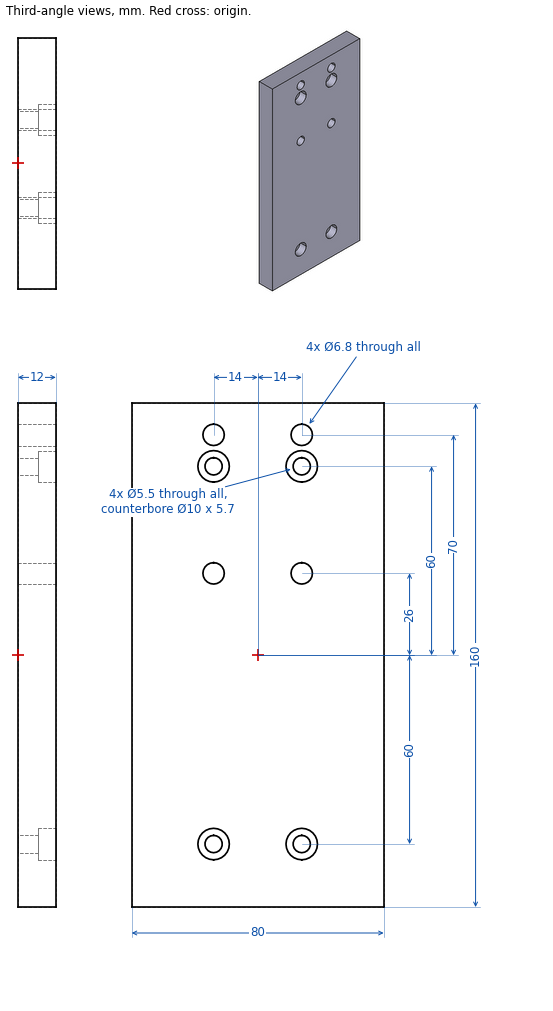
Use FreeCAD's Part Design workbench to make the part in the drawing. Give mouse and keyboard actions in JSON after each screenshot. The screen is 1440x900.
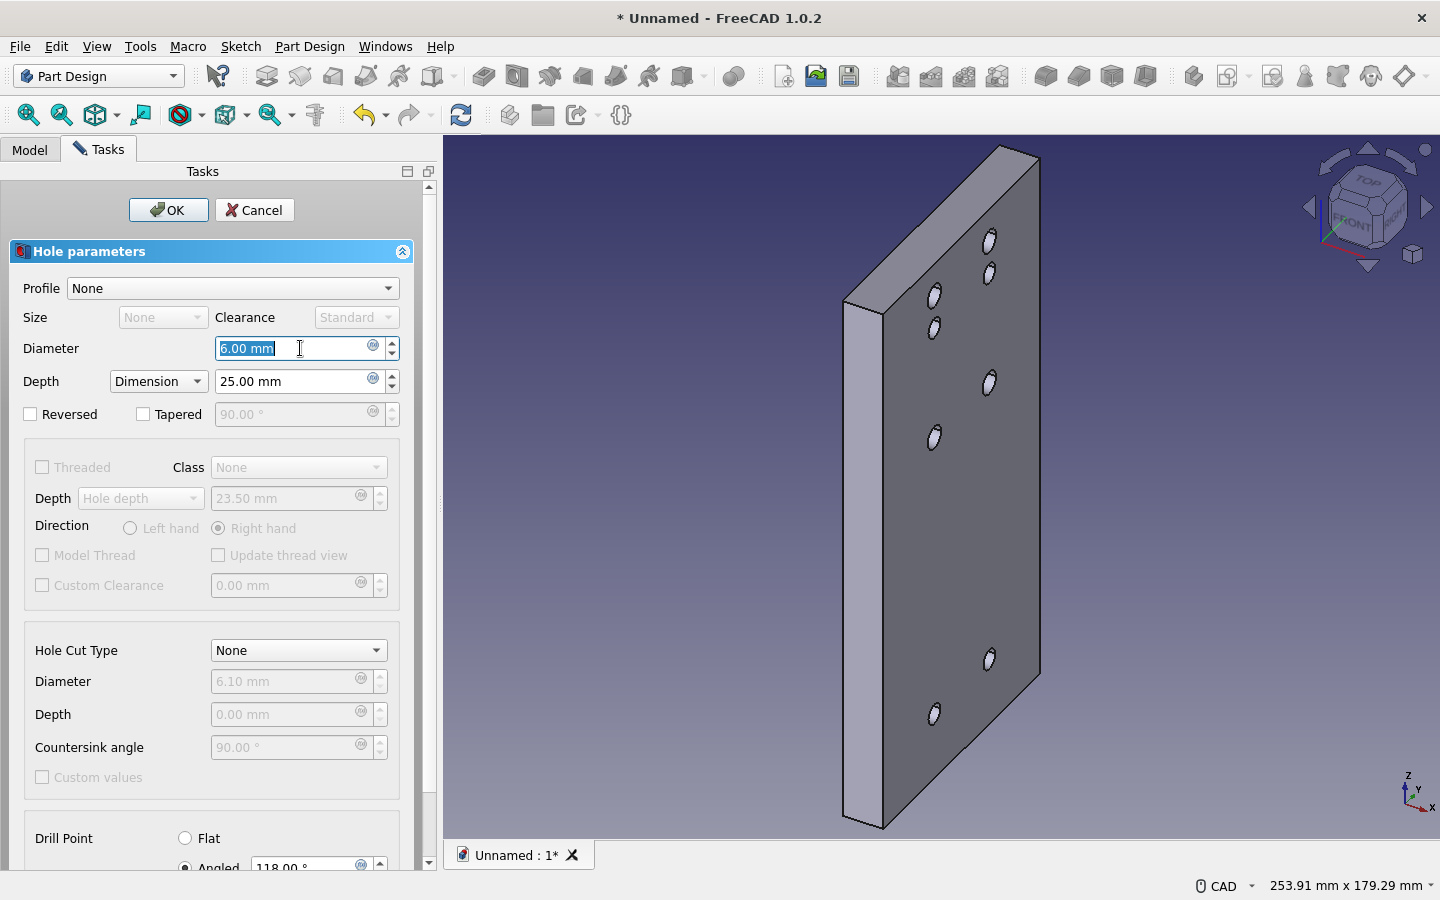
{"action": "type", "text": "5.5"}
{"action": "key", "text": "Tab"}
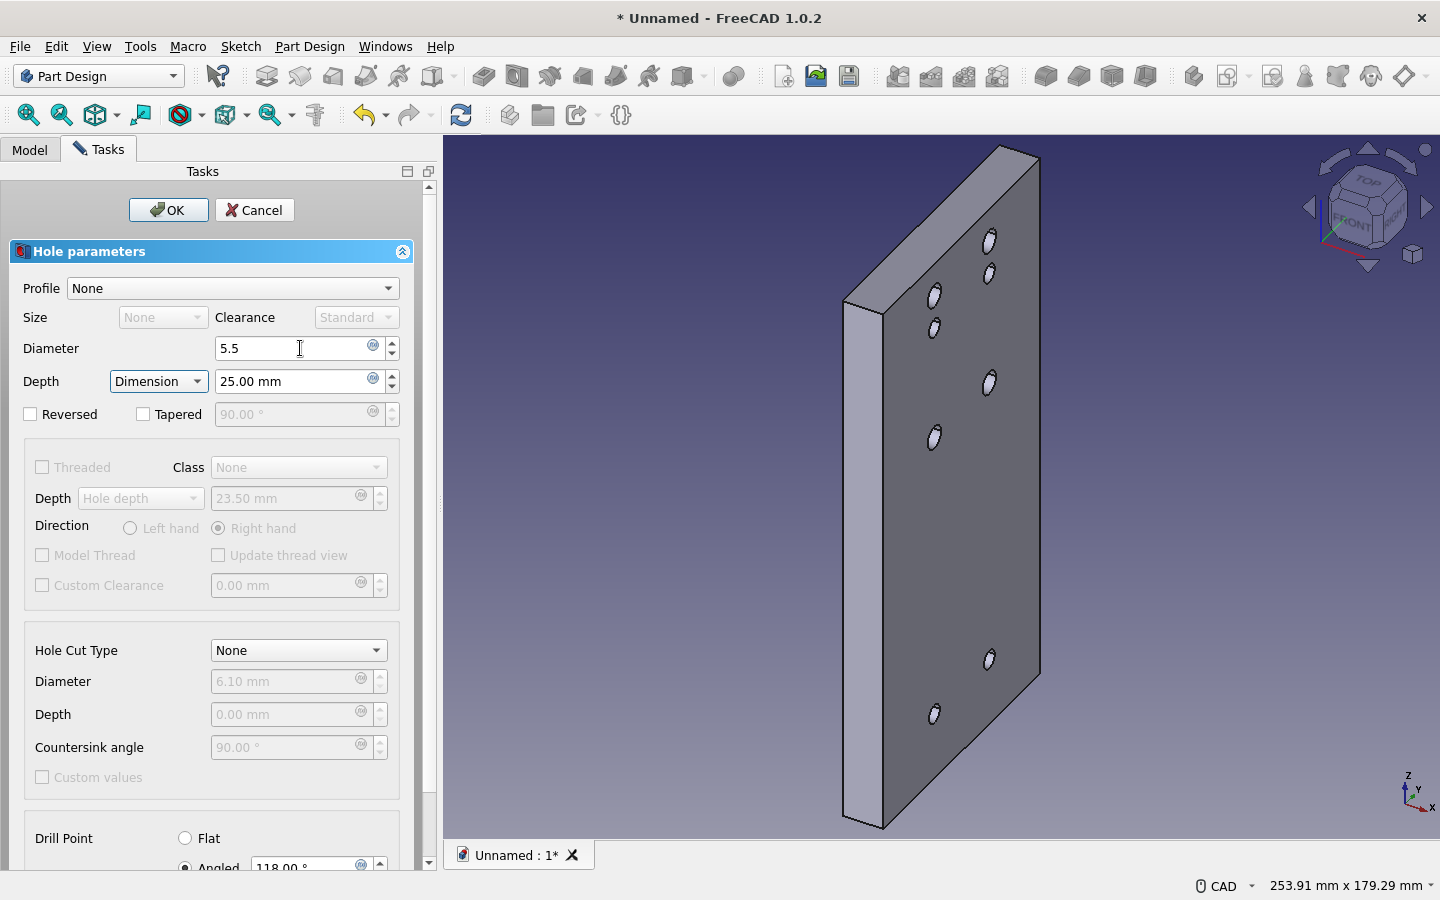
{"action": "left_click", "coordinate": [160, 382]}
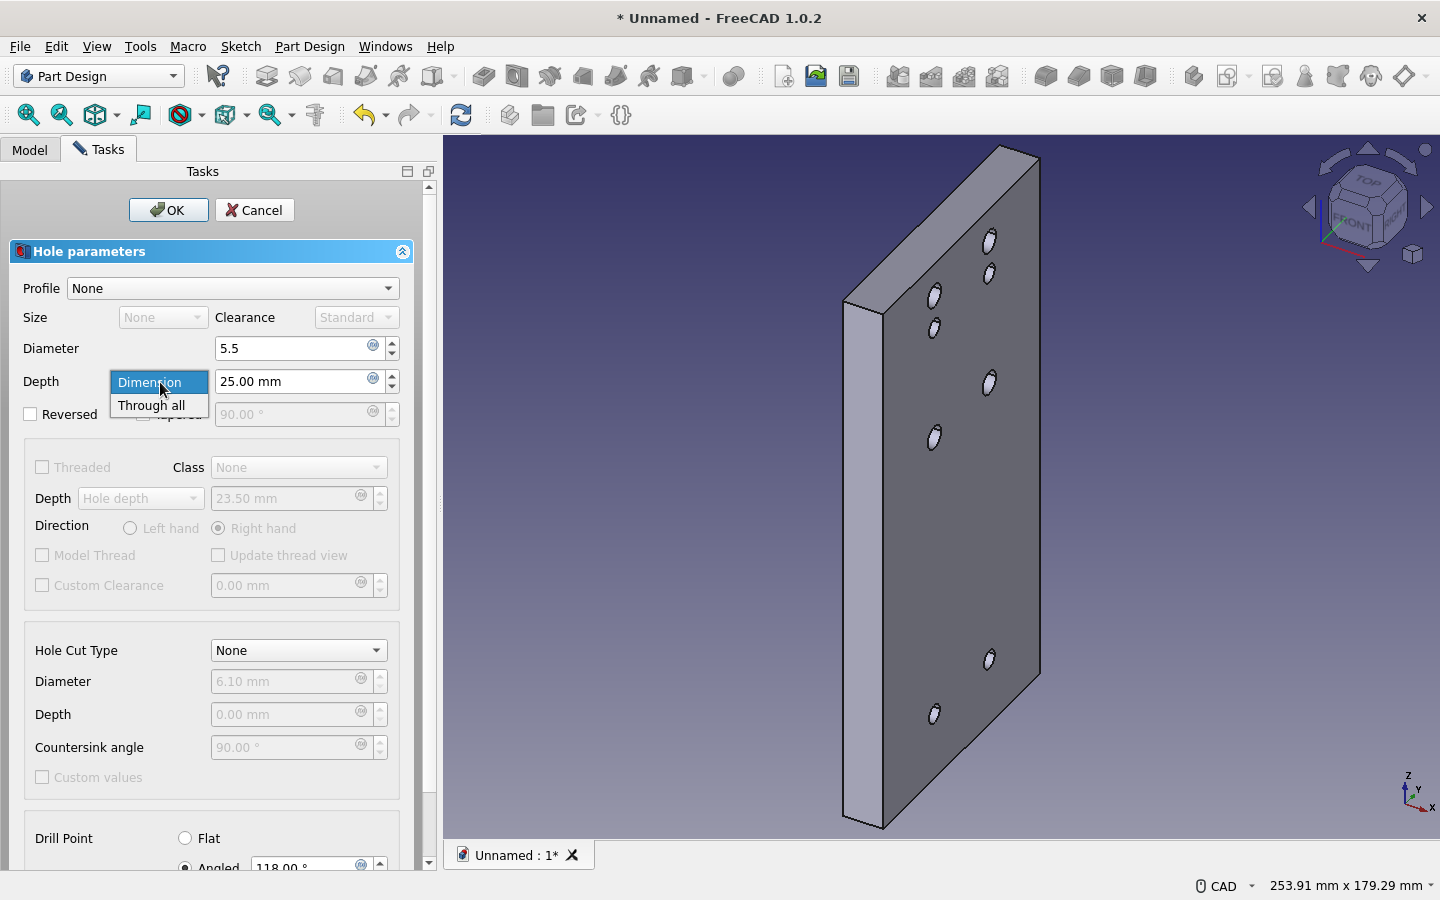
{"action": "left_click", "coordinate": [158, 406]}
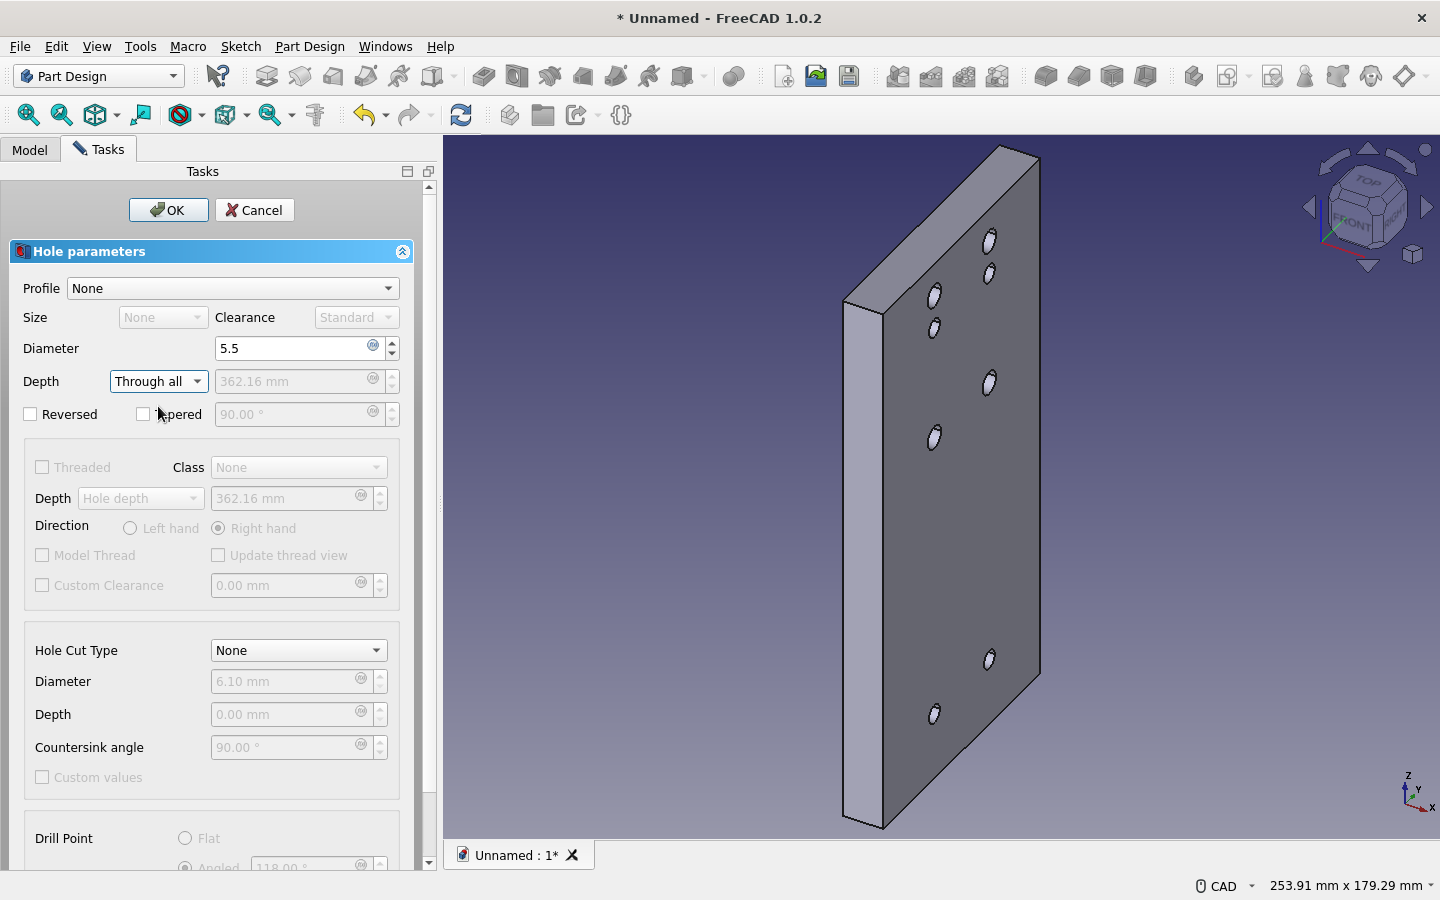
{"action": "left_click", "coordinate": [300, 650]}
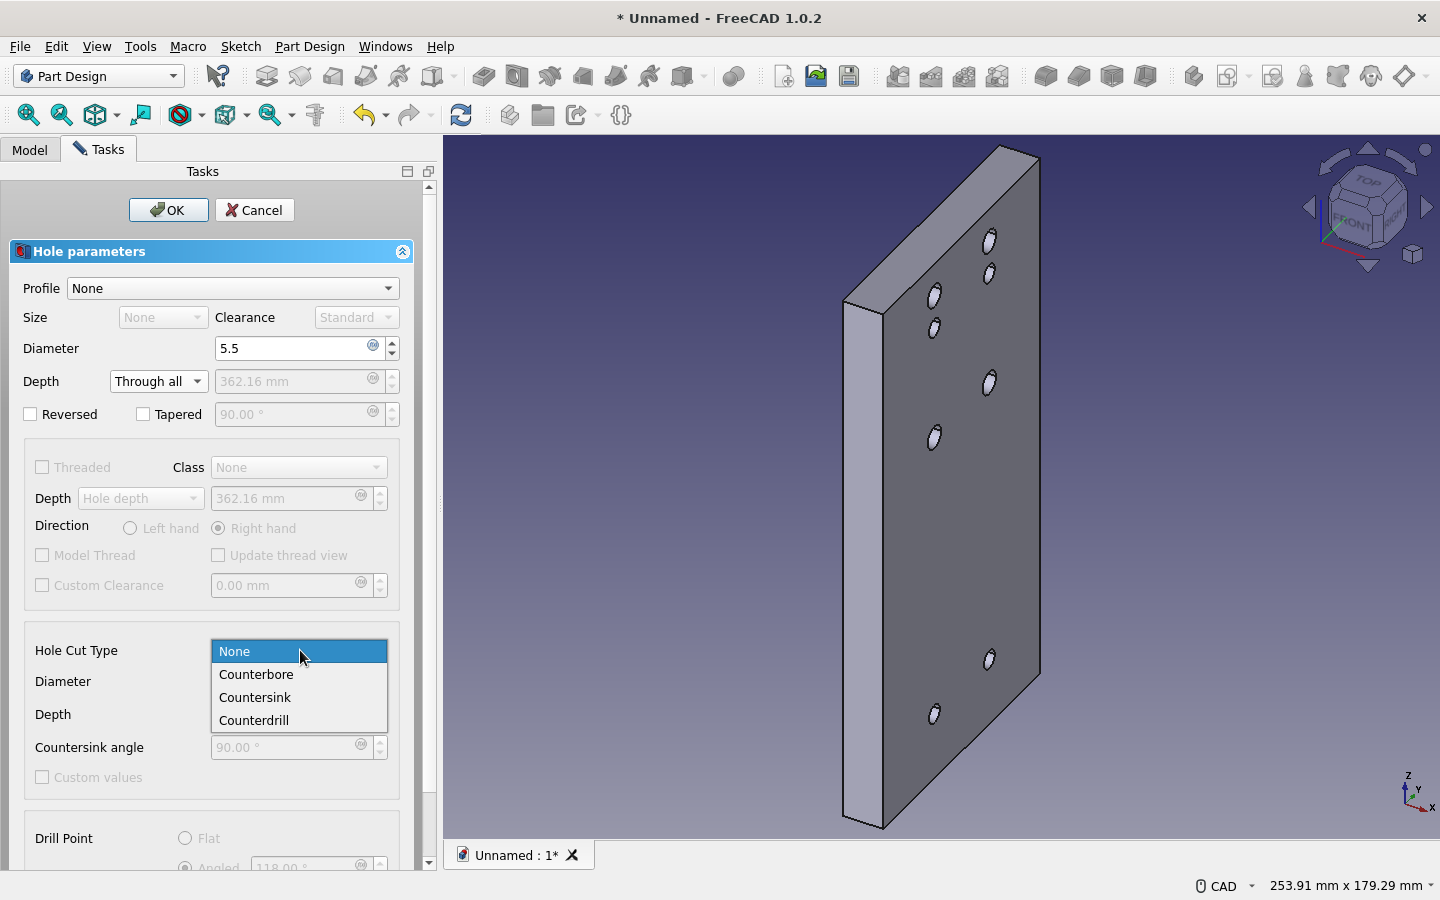
{"action": "left_click", "coordinate": [298, 674]}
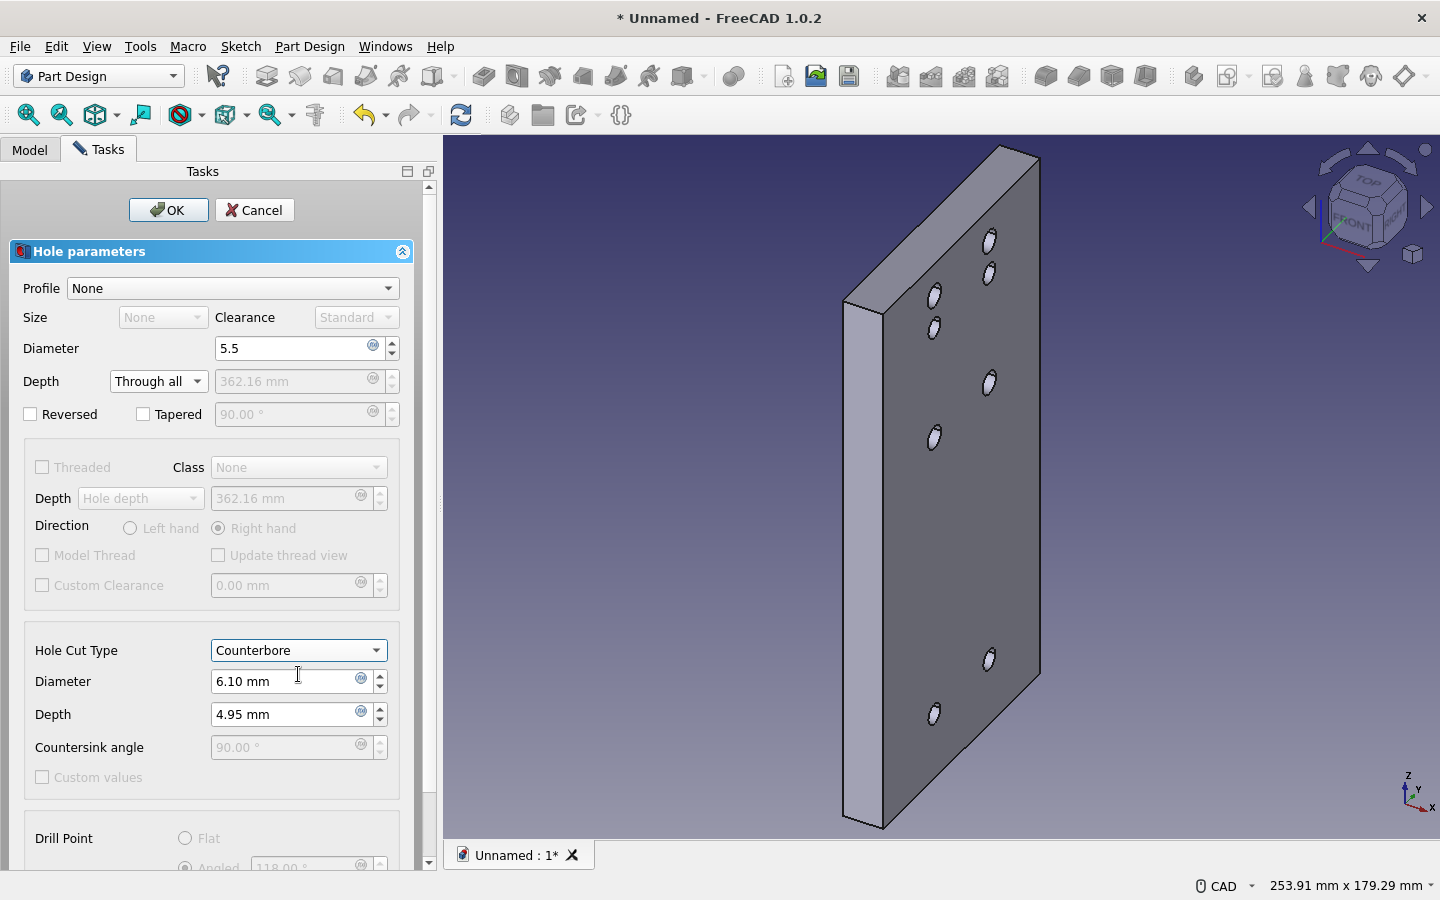
{"action": "triple_click", "coordinate": [292, 682]}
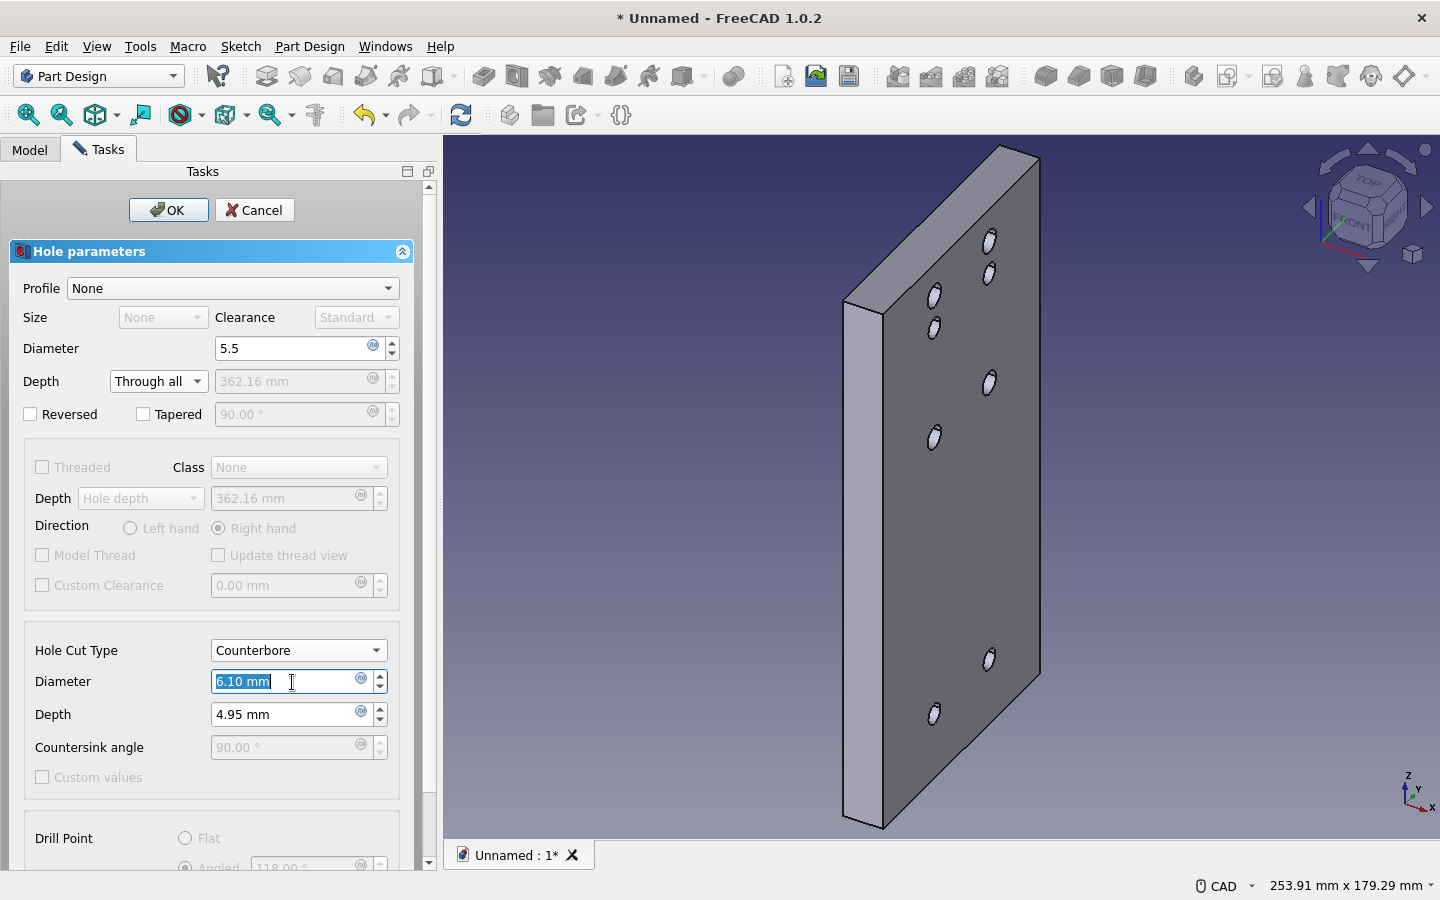
{"action": "type", "text": "10"}
{"action": "key", "text": "Tab"}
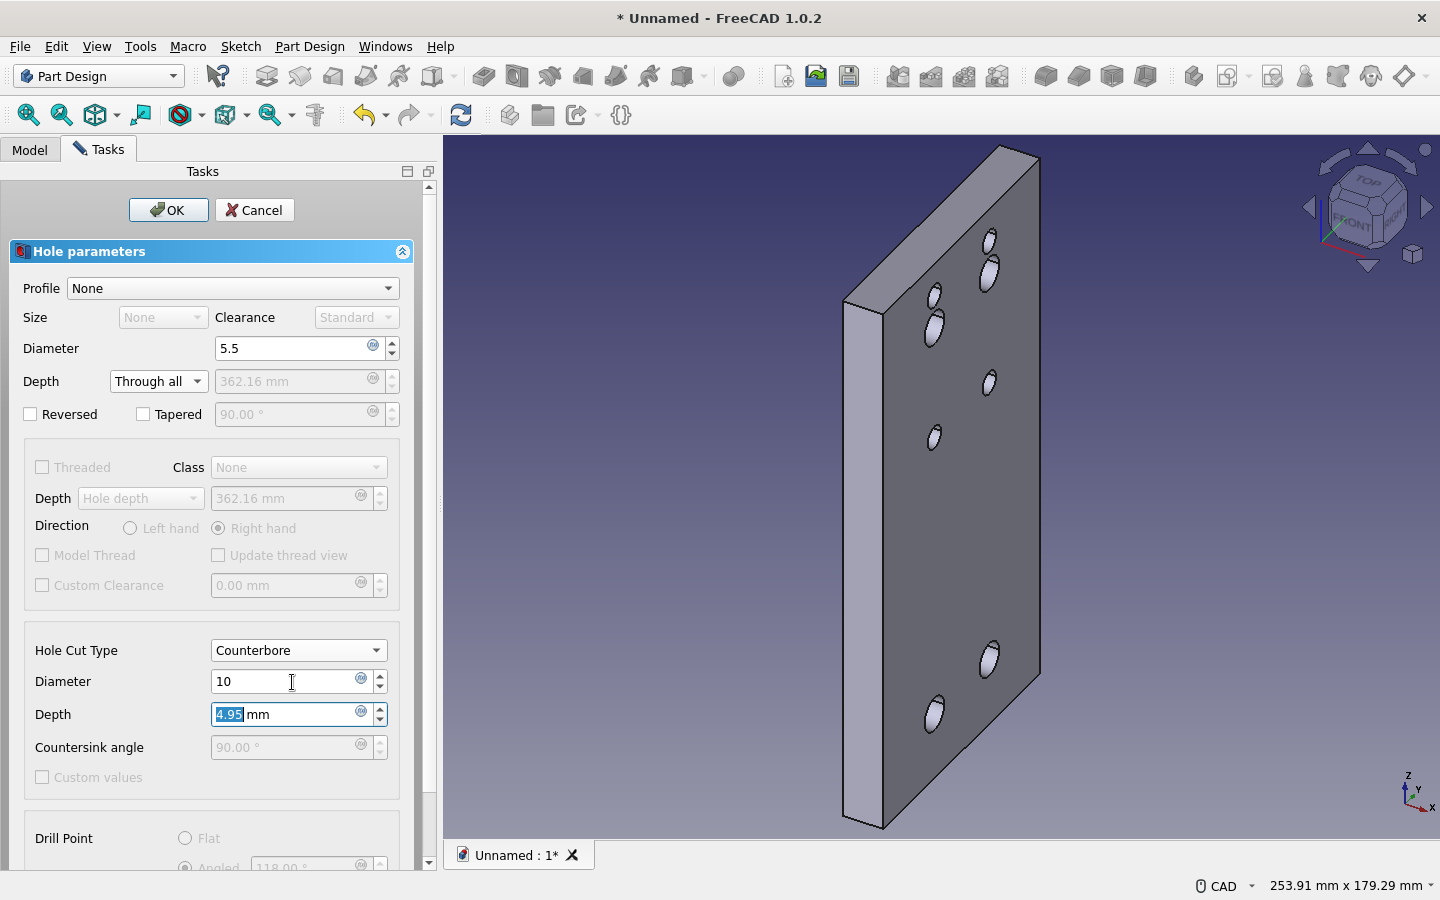
{"action": "type", "text": "5.7"}
{"action": "key", "text": "Tab"}